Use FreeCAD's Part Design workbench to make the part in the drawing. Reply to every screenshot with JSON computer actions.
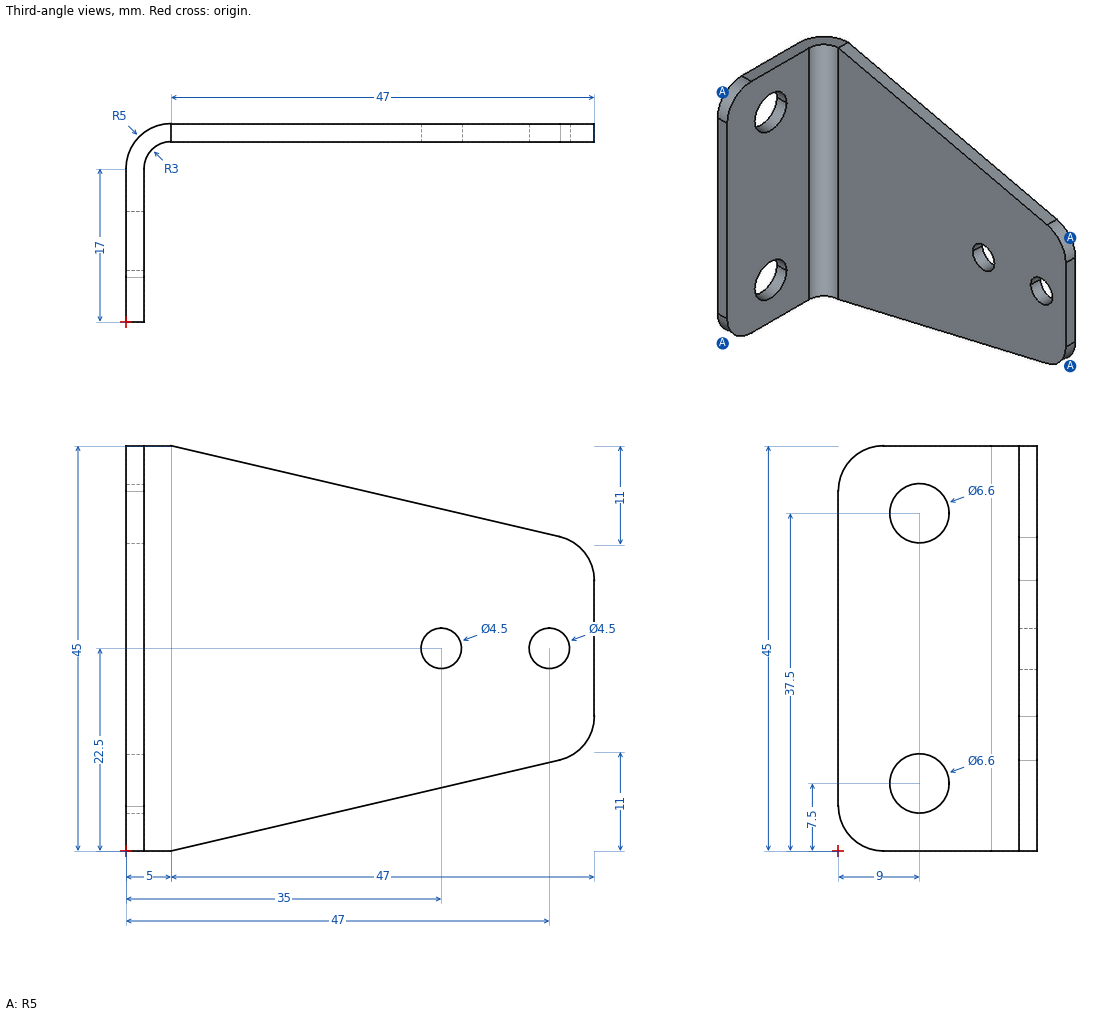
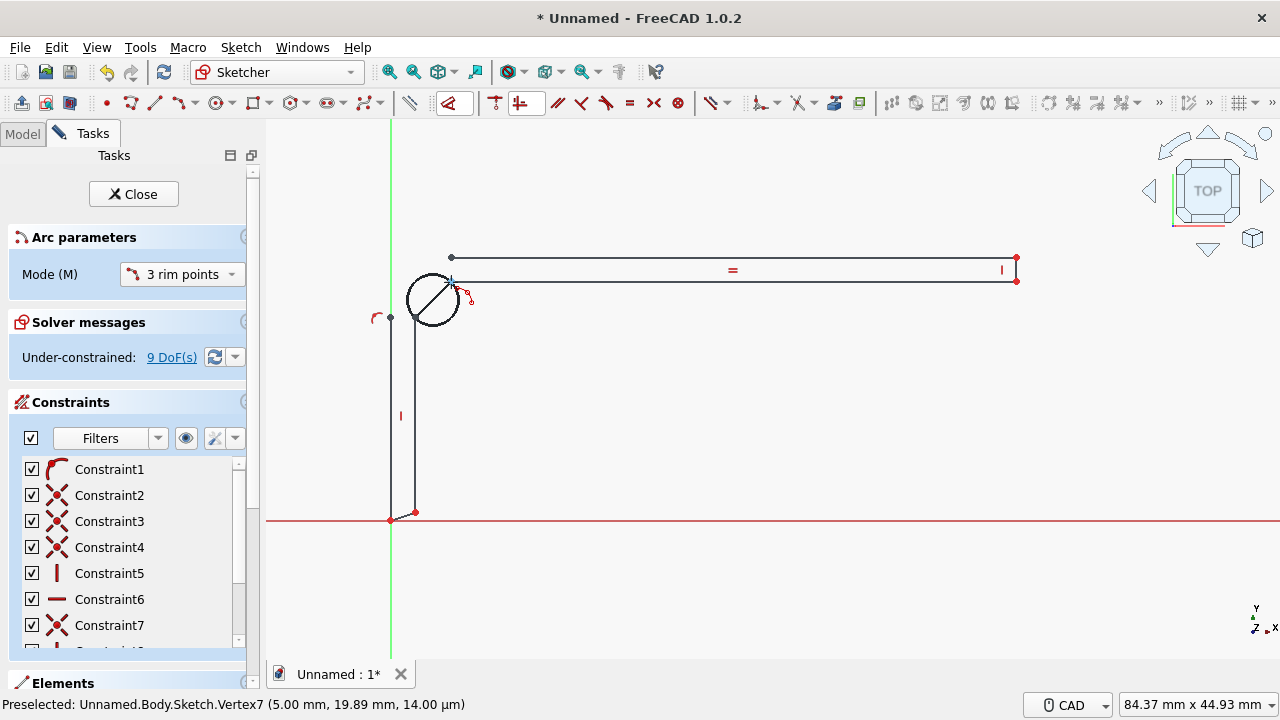
{"action": "scroll", "coordinate": [425, 291], "scroll_direction": "up", "scroll_amount": 3}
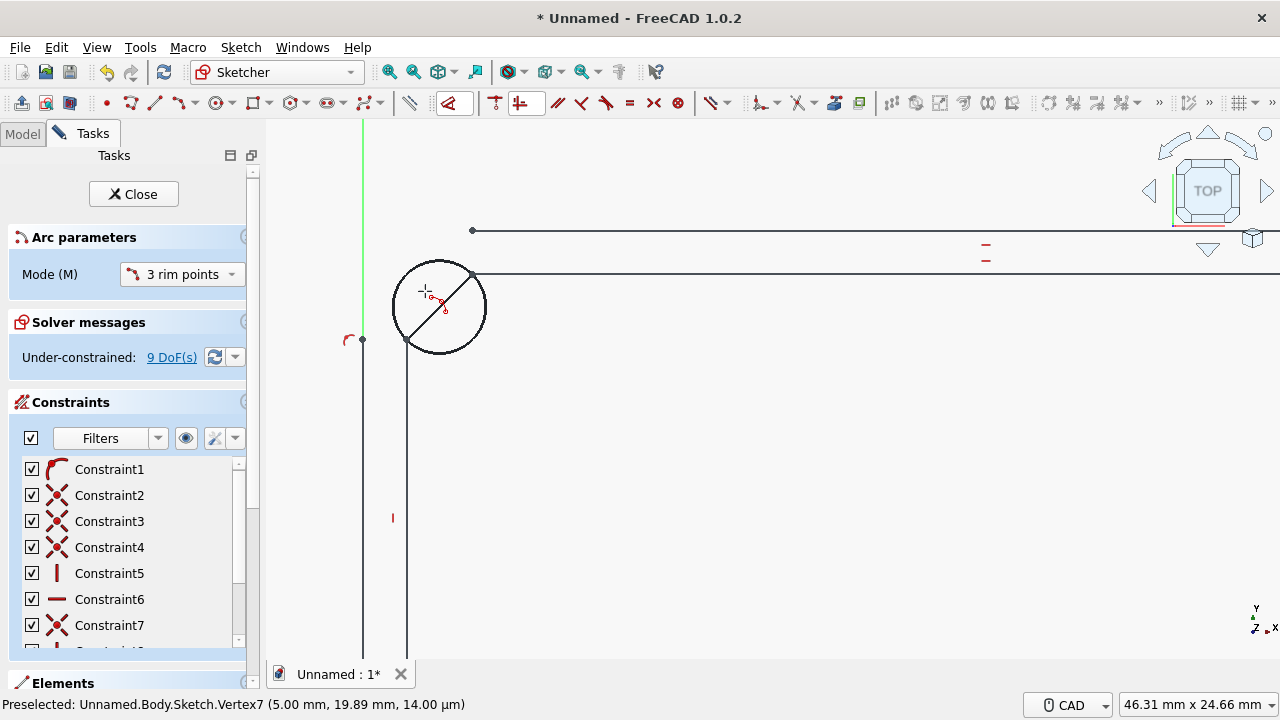
{"action": "left_click", "coordinate": [426, 291]}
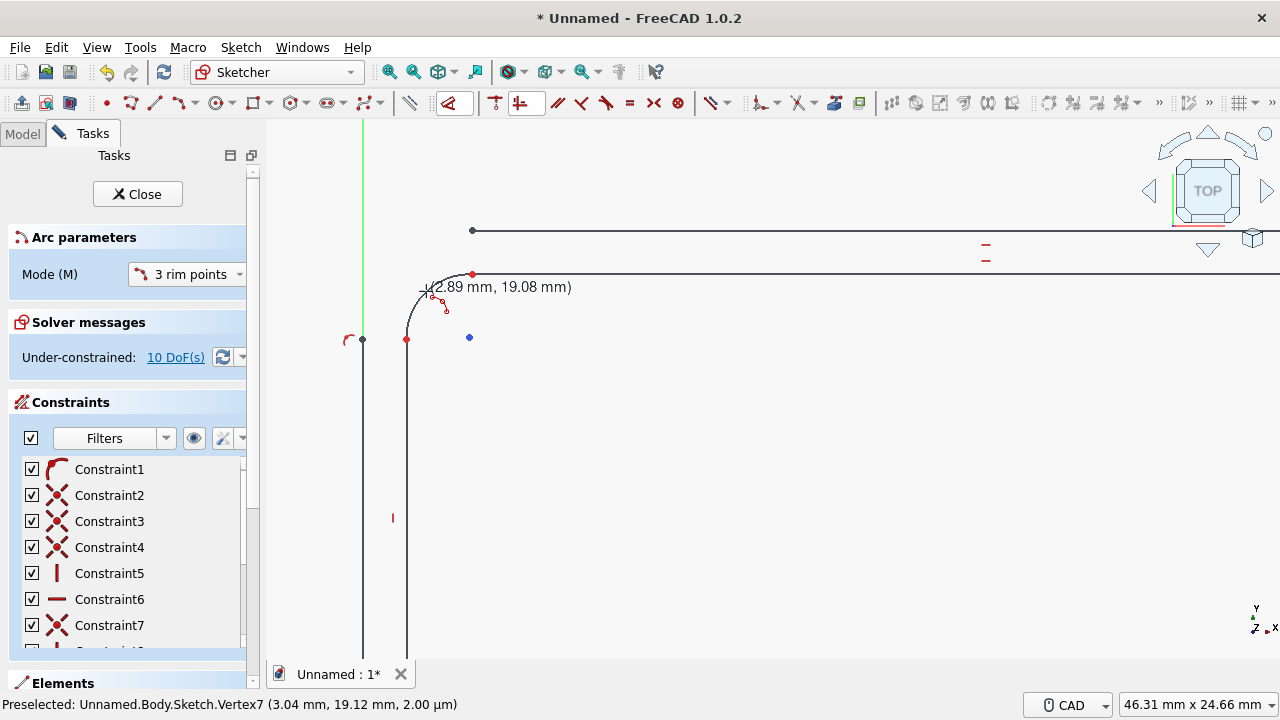
{"action": "left_click", "coordinate": [472, 231]}
{"action": "left_click", "coordinate": [363, 340]}
{"action": "left_click", "coordinate": [395, 260]}
{"action": "key", "text": "Escape"}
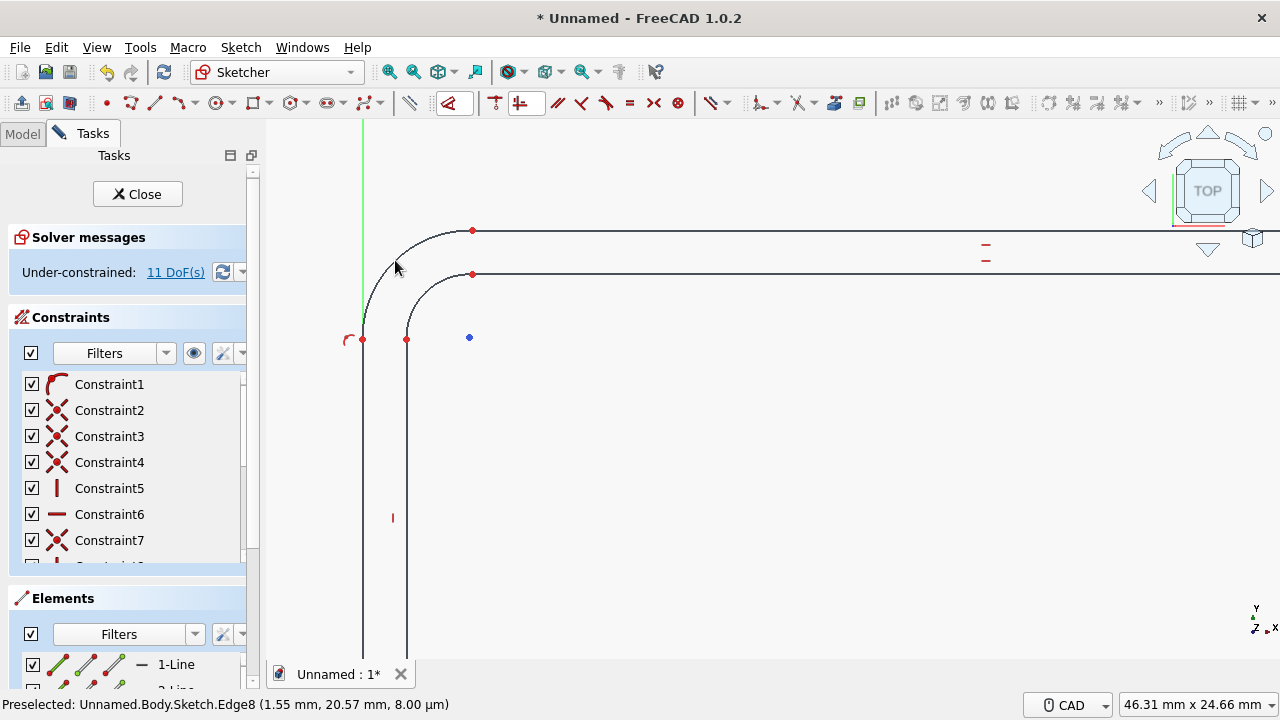
{"action": "left_click", "coordinate": [363, 451]}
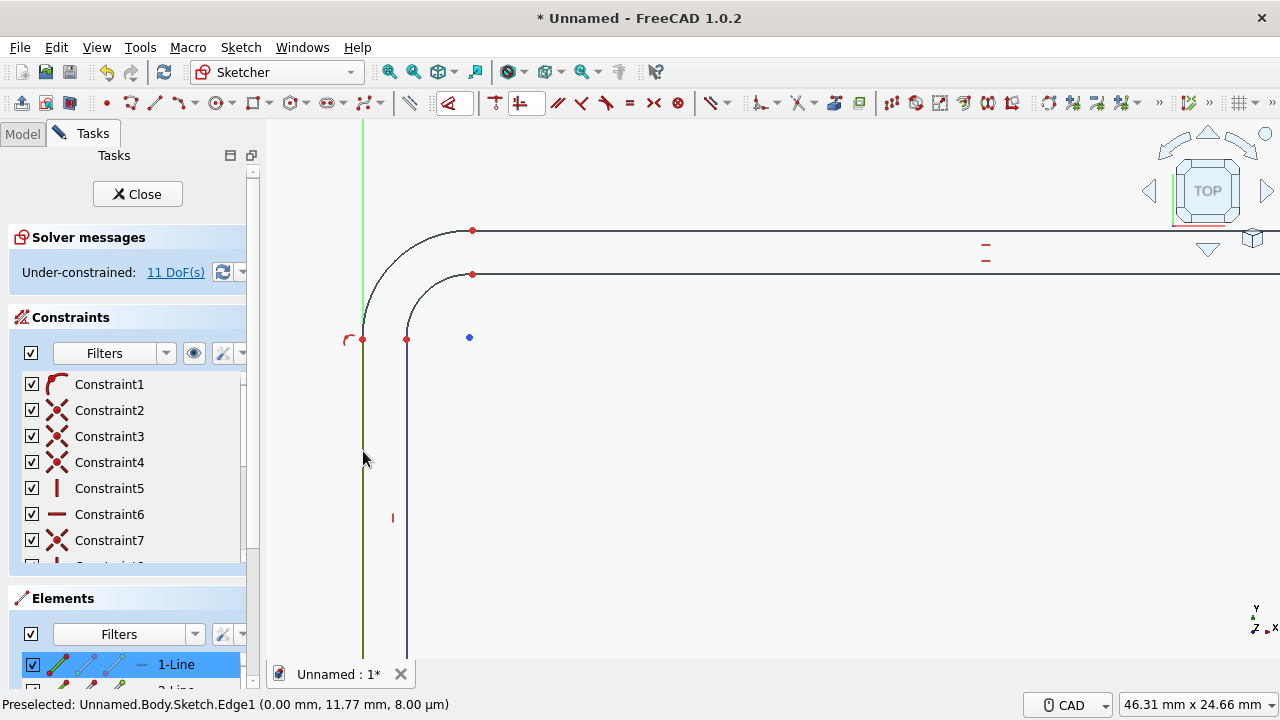
{"action": "left_click", "coordinate": [422, 242]}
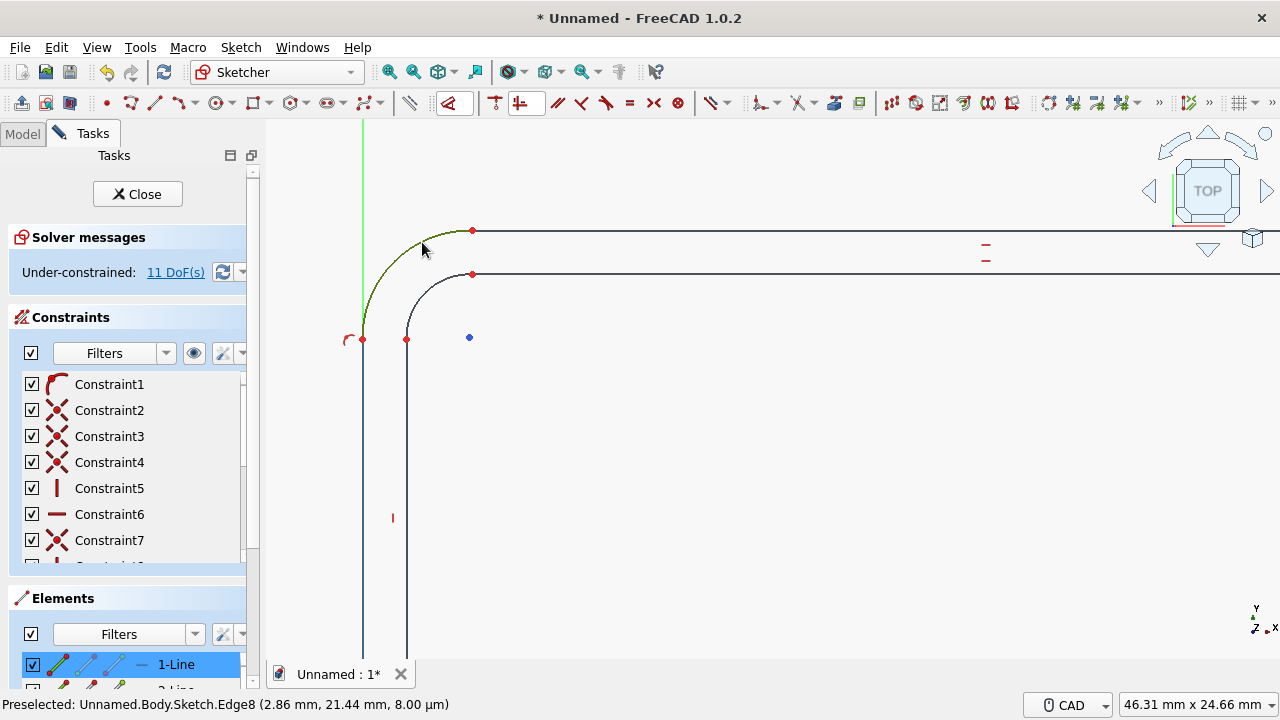
{"action": "key", "text": "t"}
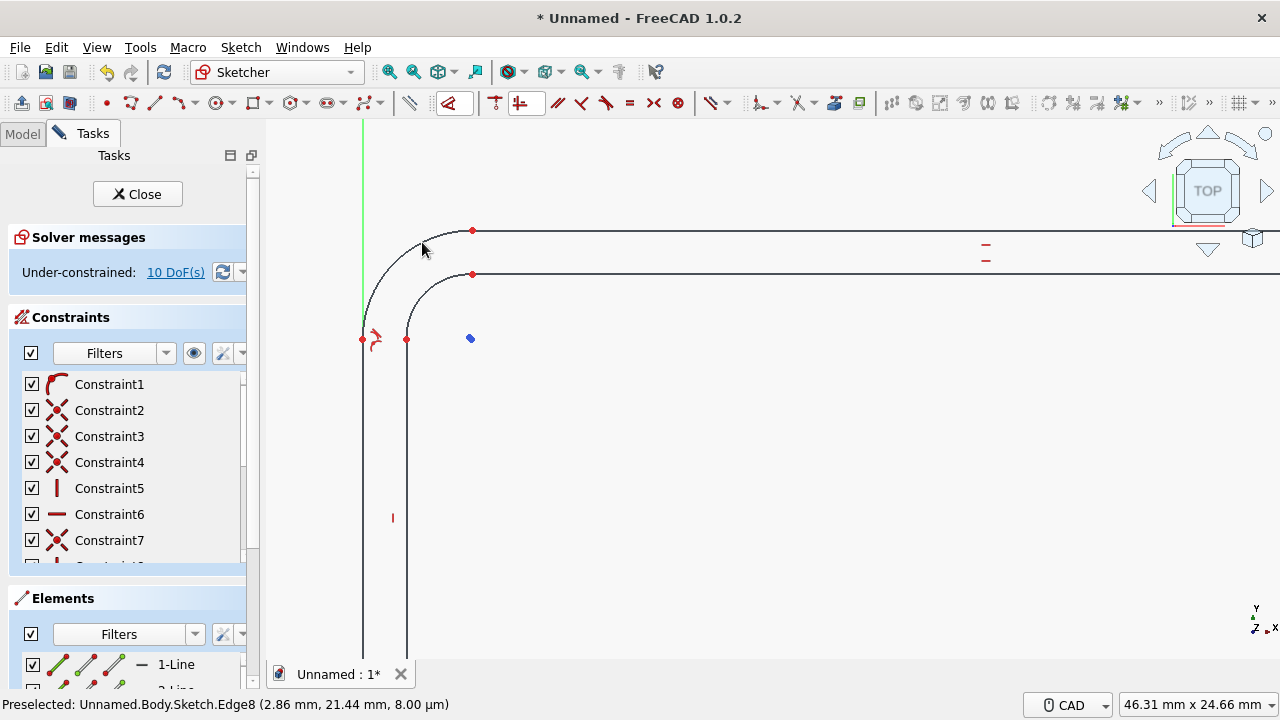
{"action": "left_click", "coordinate": [407, 589]}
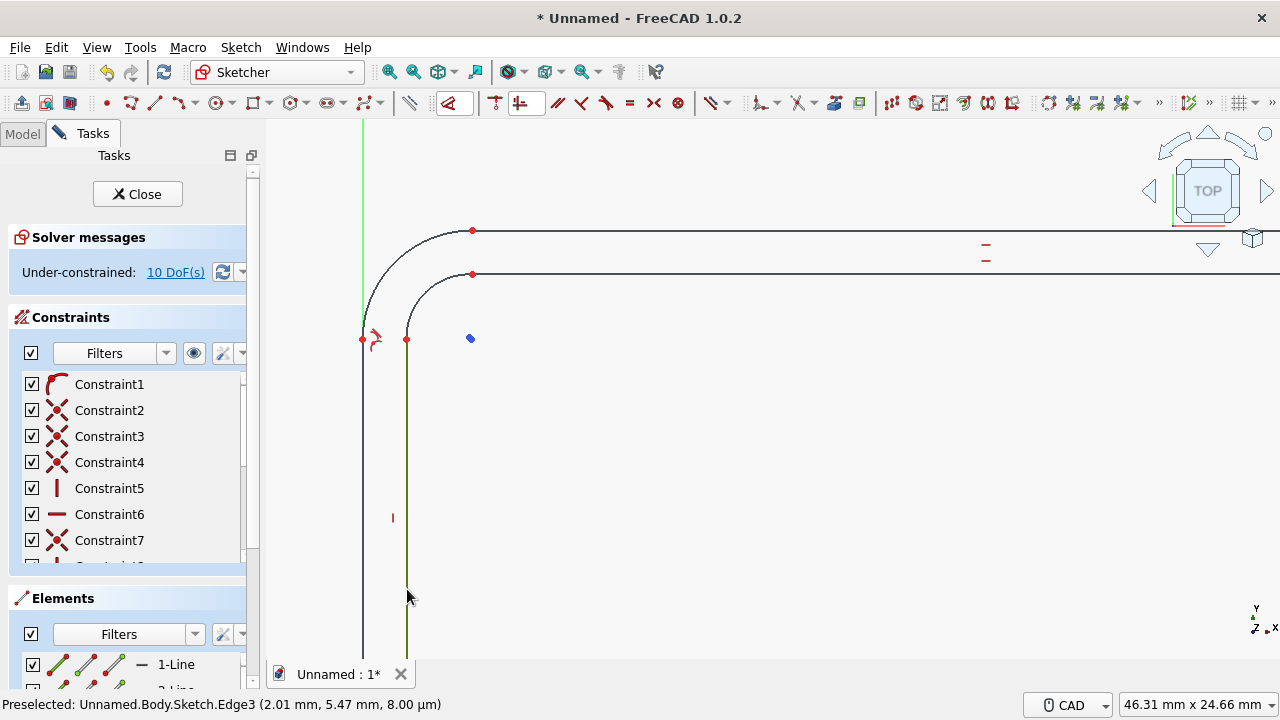
{"action": "left_click", "coordinate": [442, 281]}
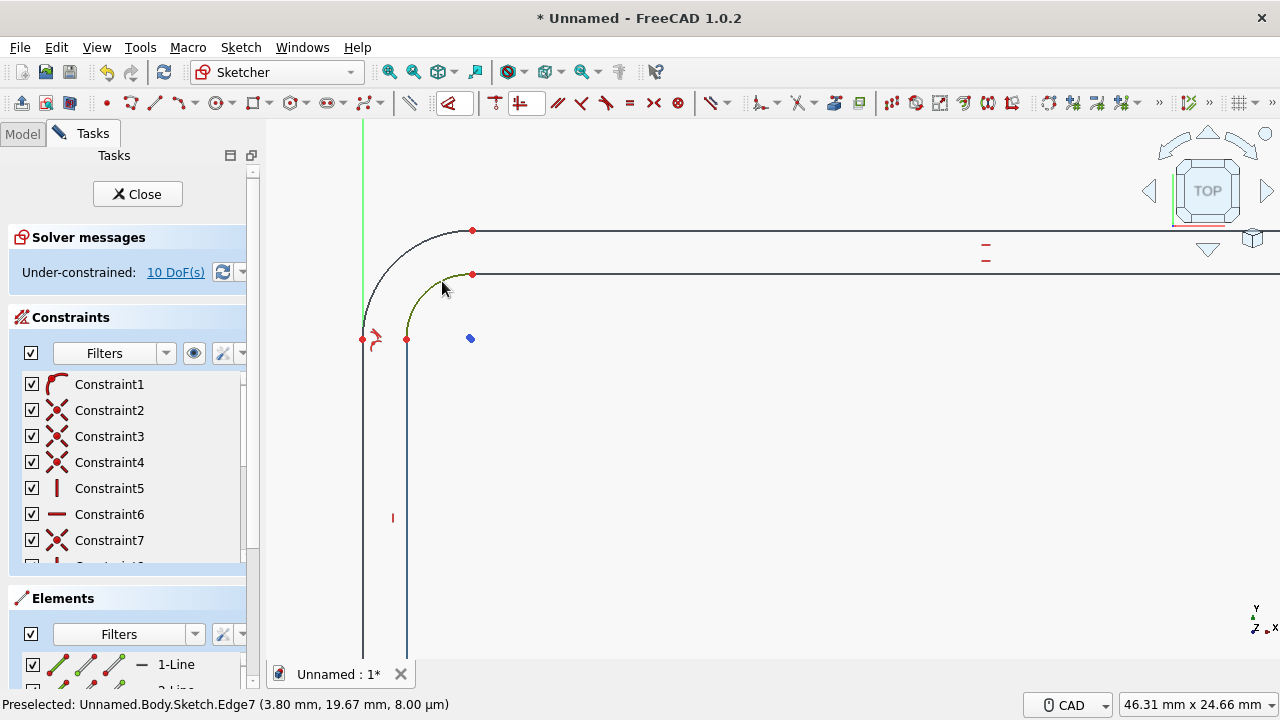
{"action": "left_click", "coordinate": [606, 104]}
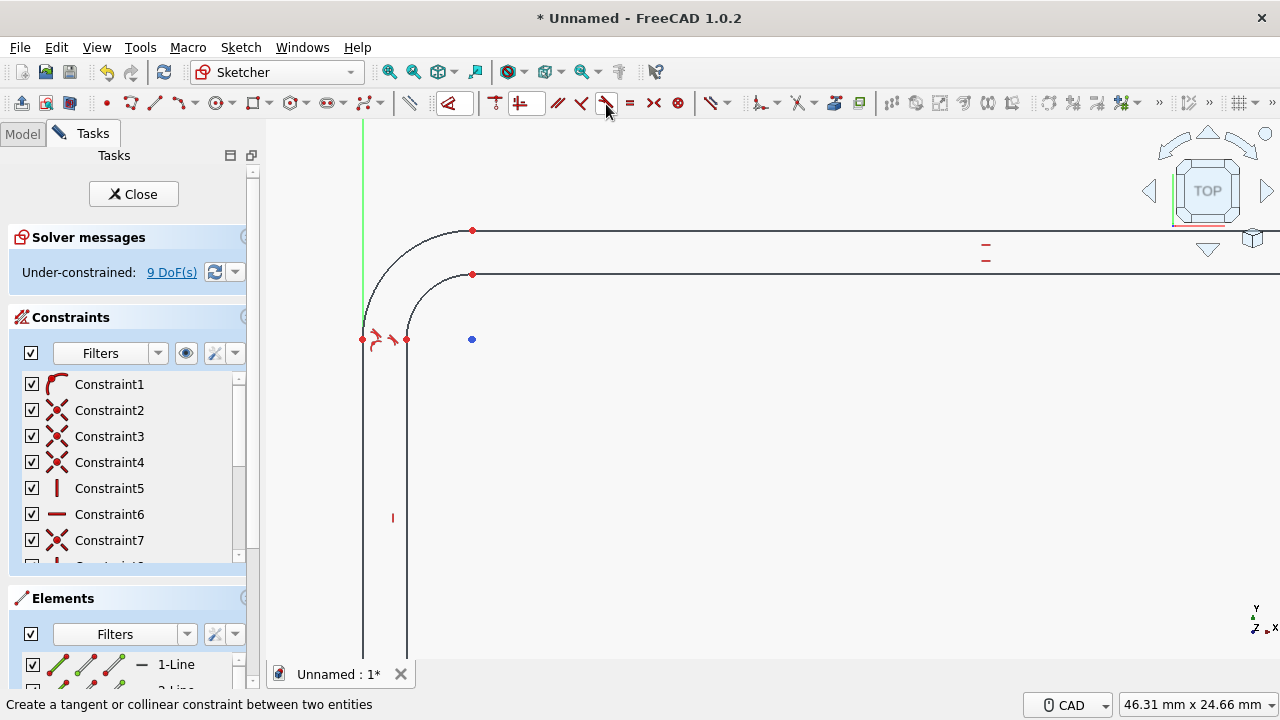
{"action": "left_click", "coordinate": [781, 274]}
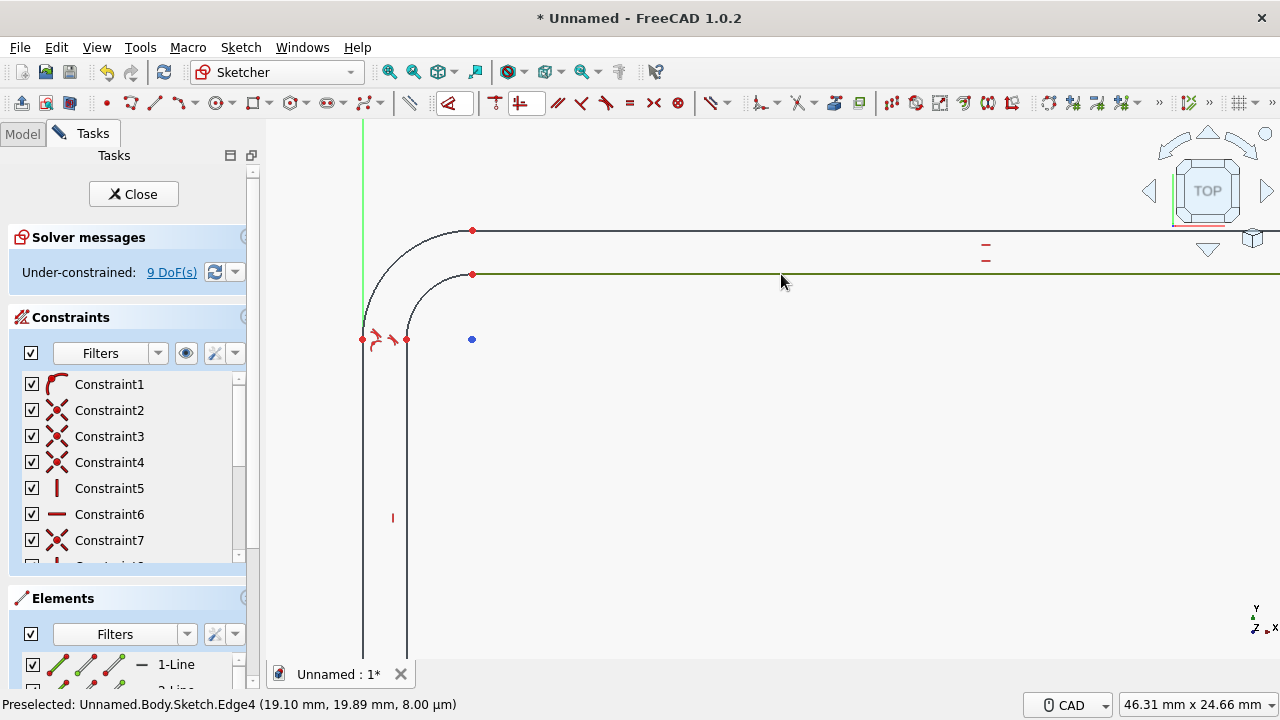
{"action": "left_click", "coordinate": [442, 281]}